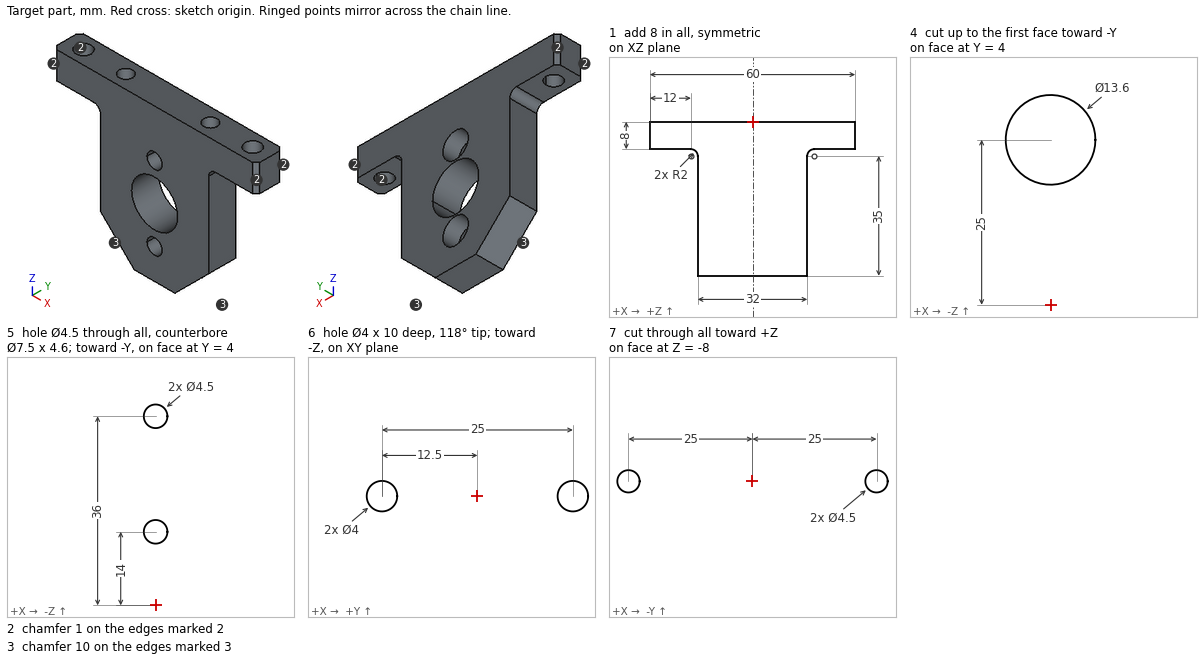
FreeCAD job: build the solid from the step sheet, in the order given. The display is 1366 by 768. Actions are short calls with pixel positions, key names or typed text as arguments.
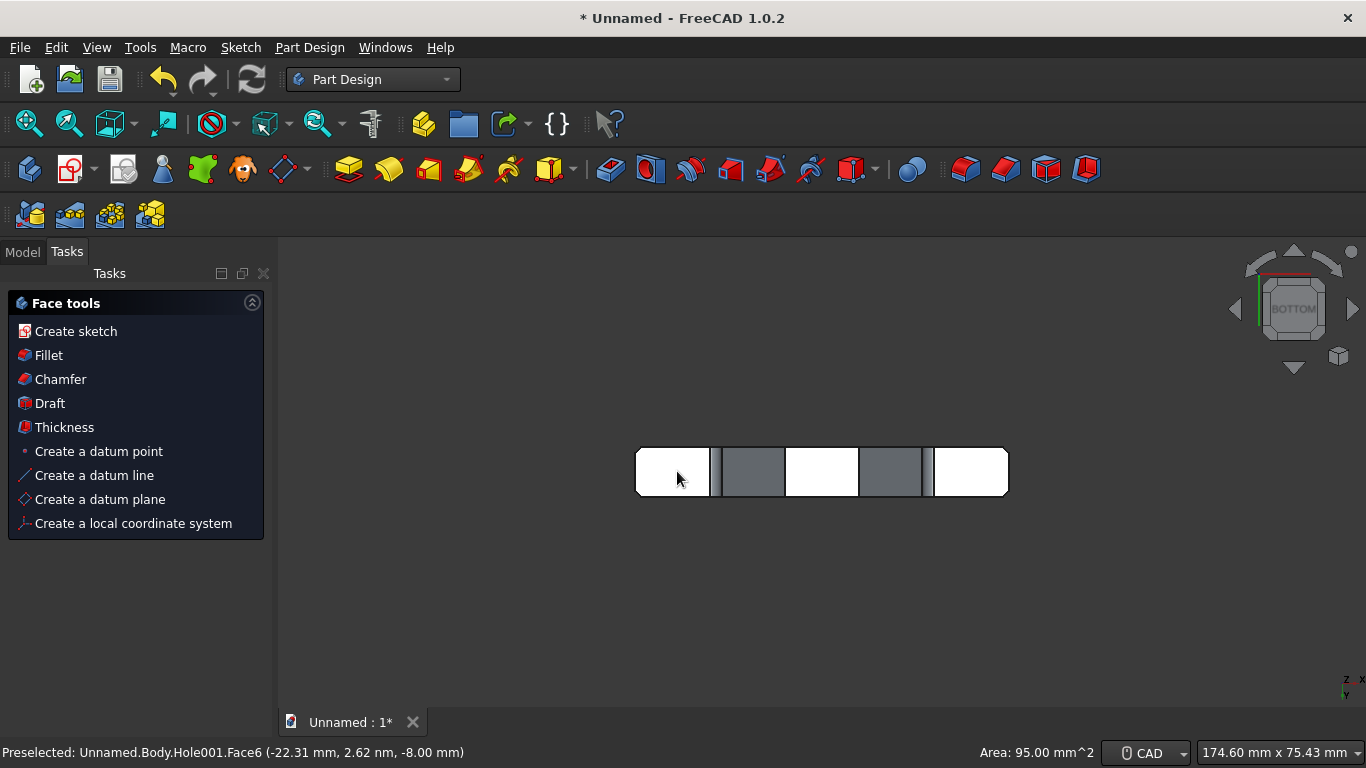
click(70, 170)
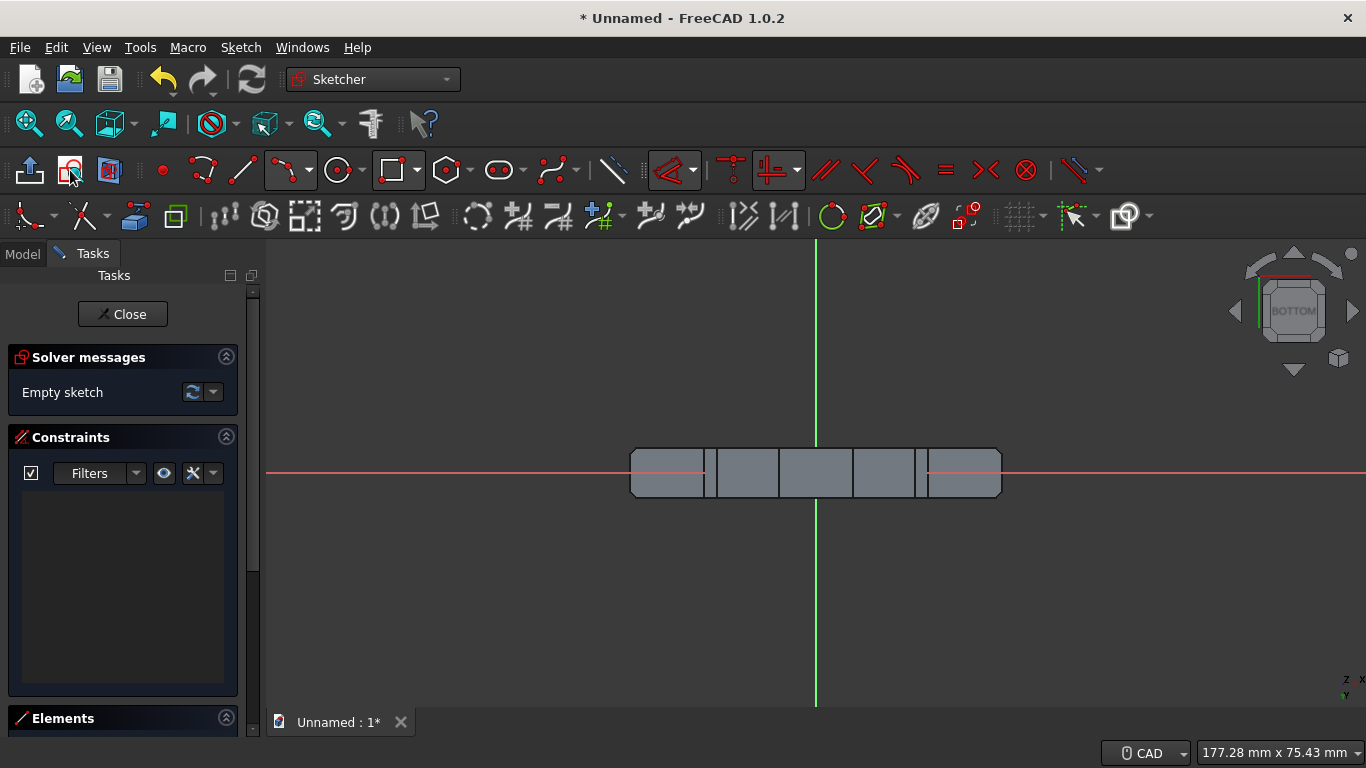
scroll(899, 473, up, 3)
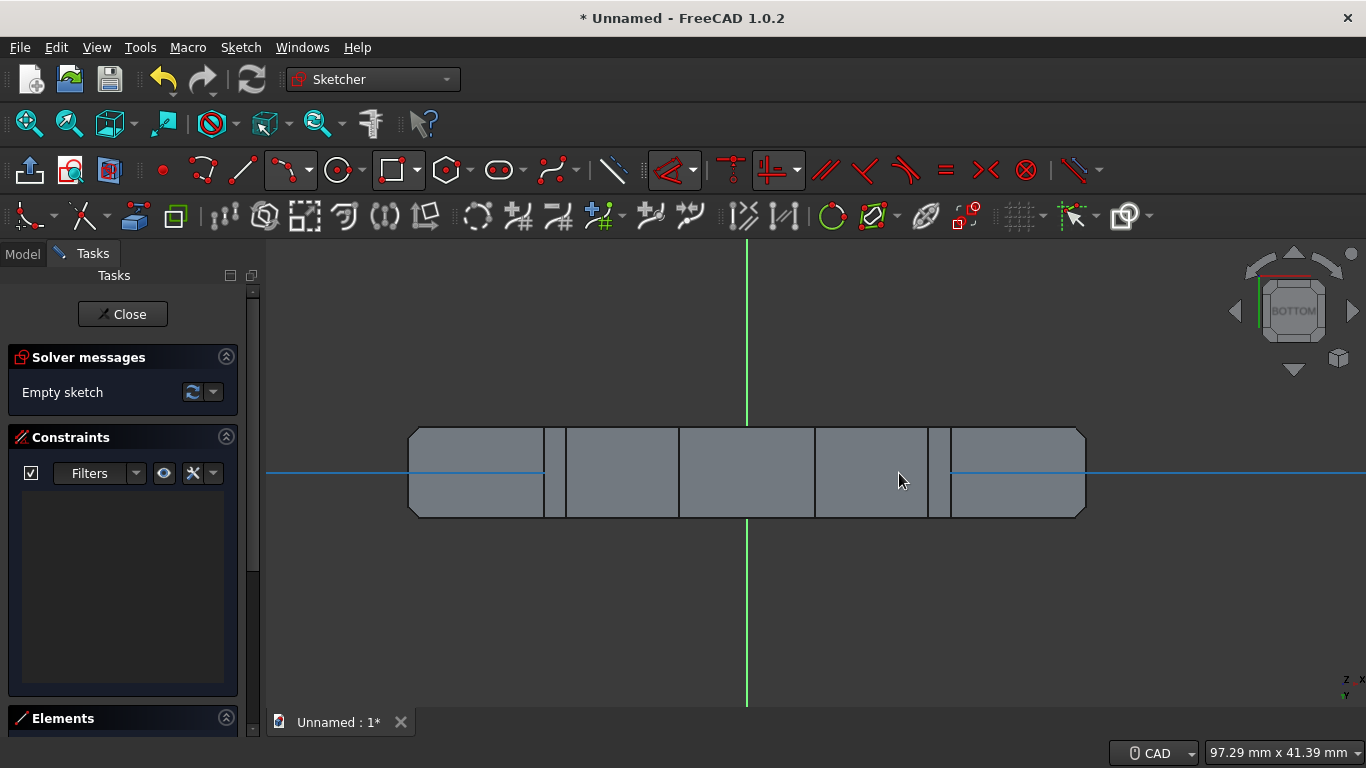
click(338, 170)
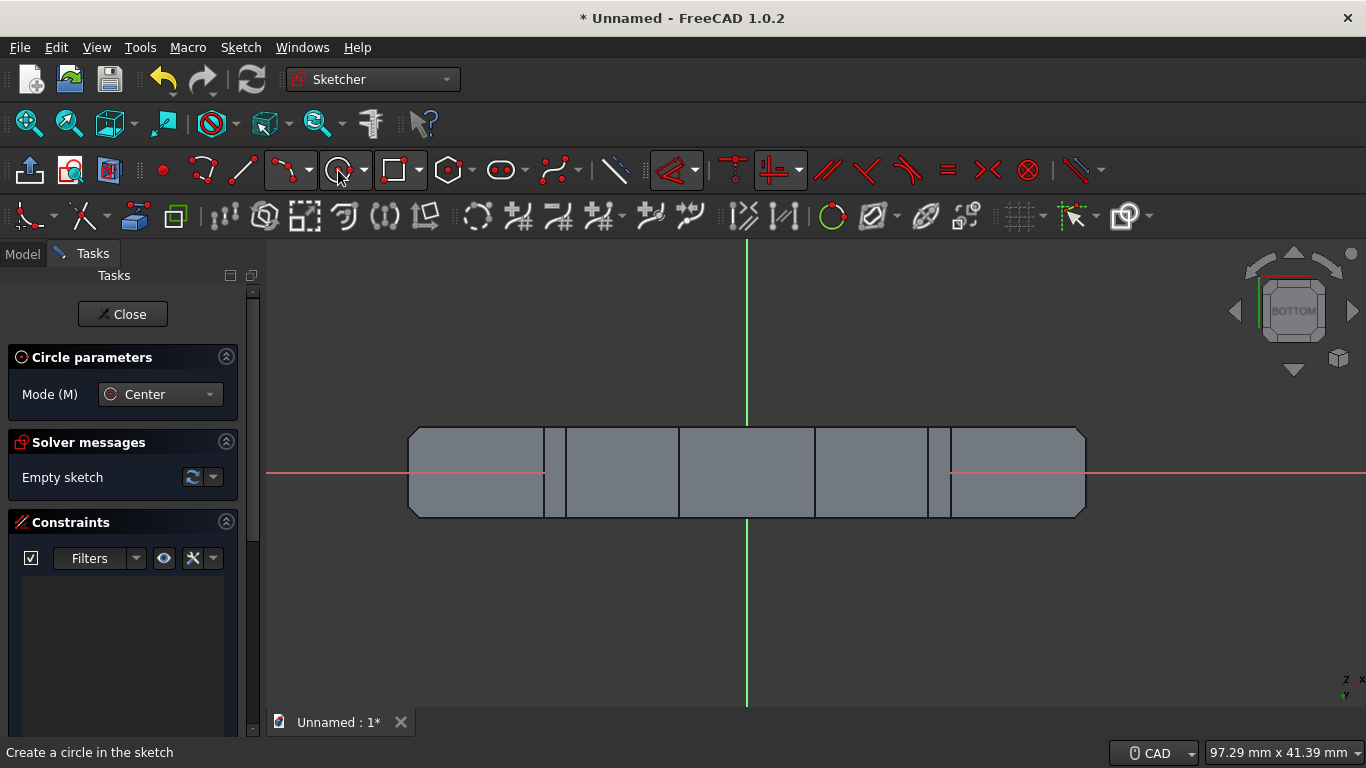
click(1030, 473)
click(1048, 455)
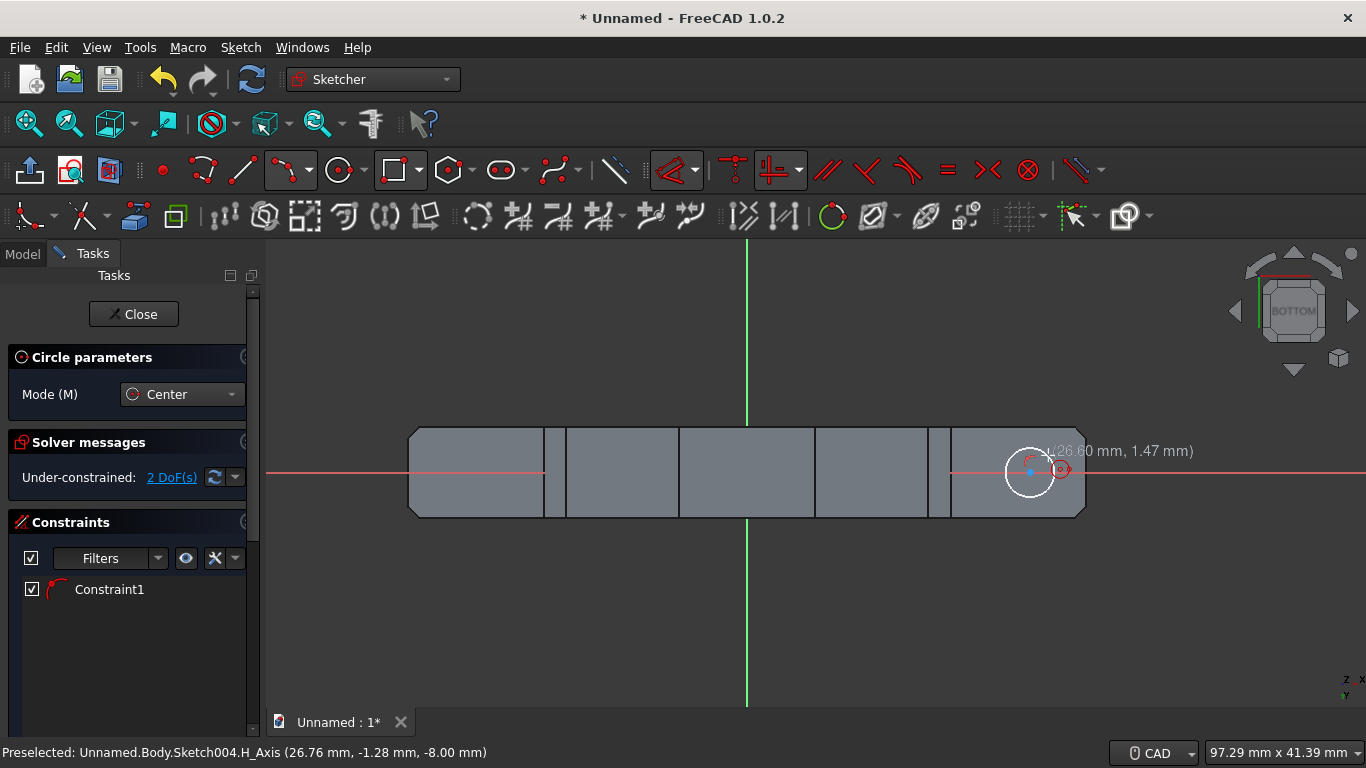
click(465, 473)
click(483, 455)
key(Escape)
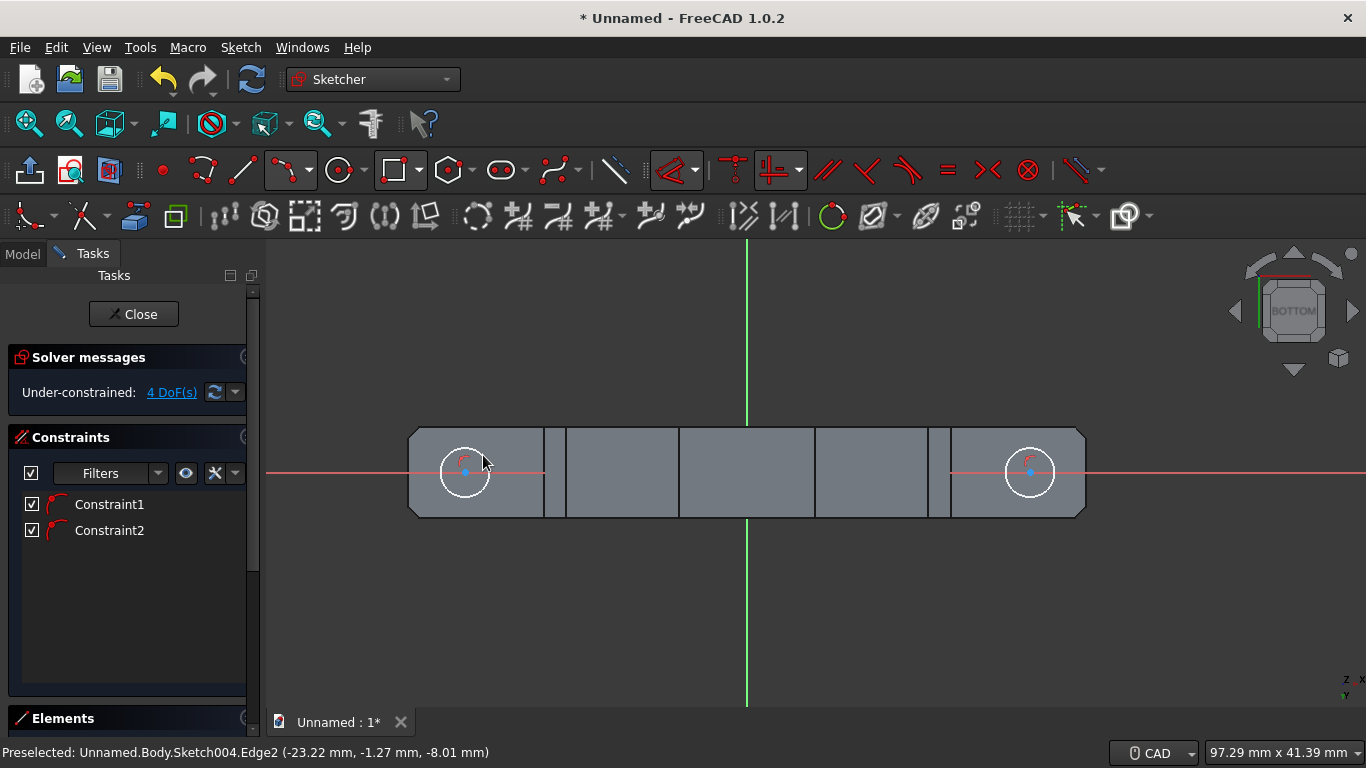
click(1047, 455)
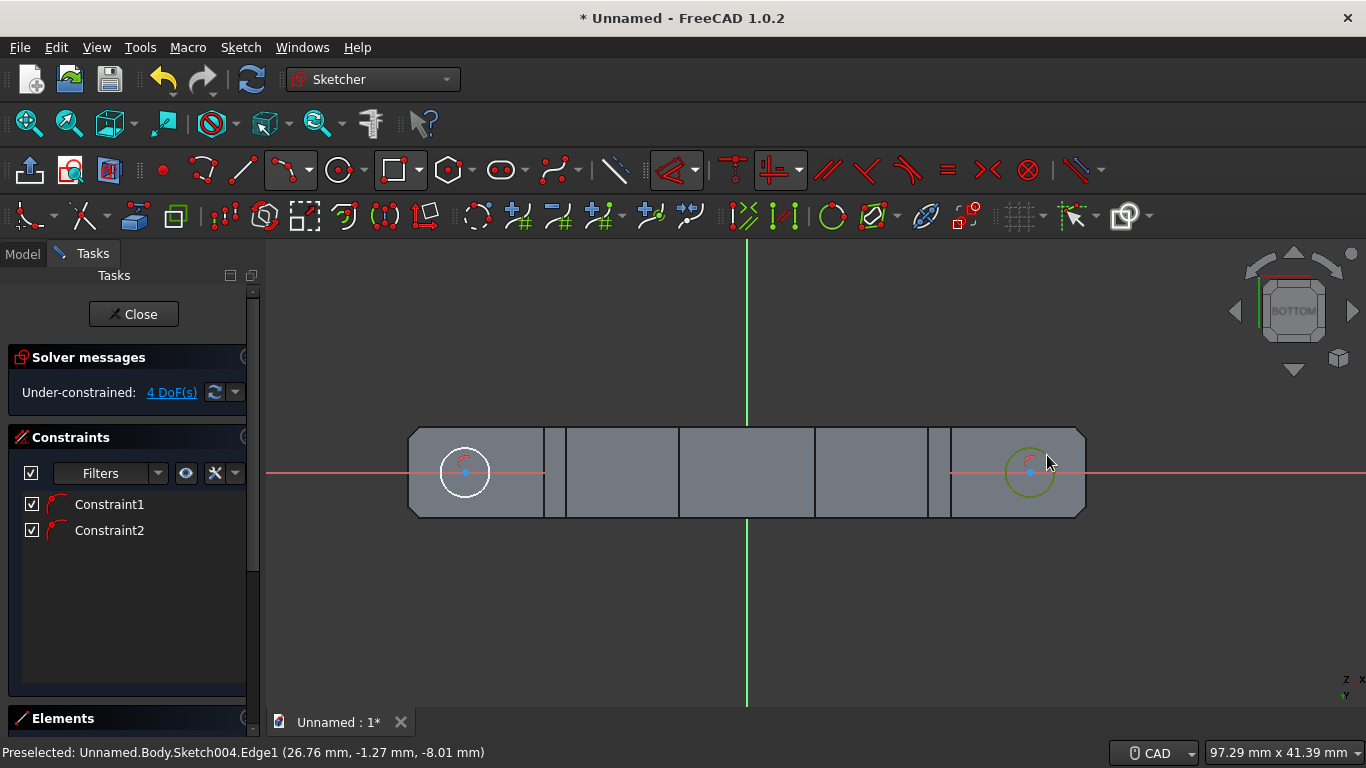
click(482, 455)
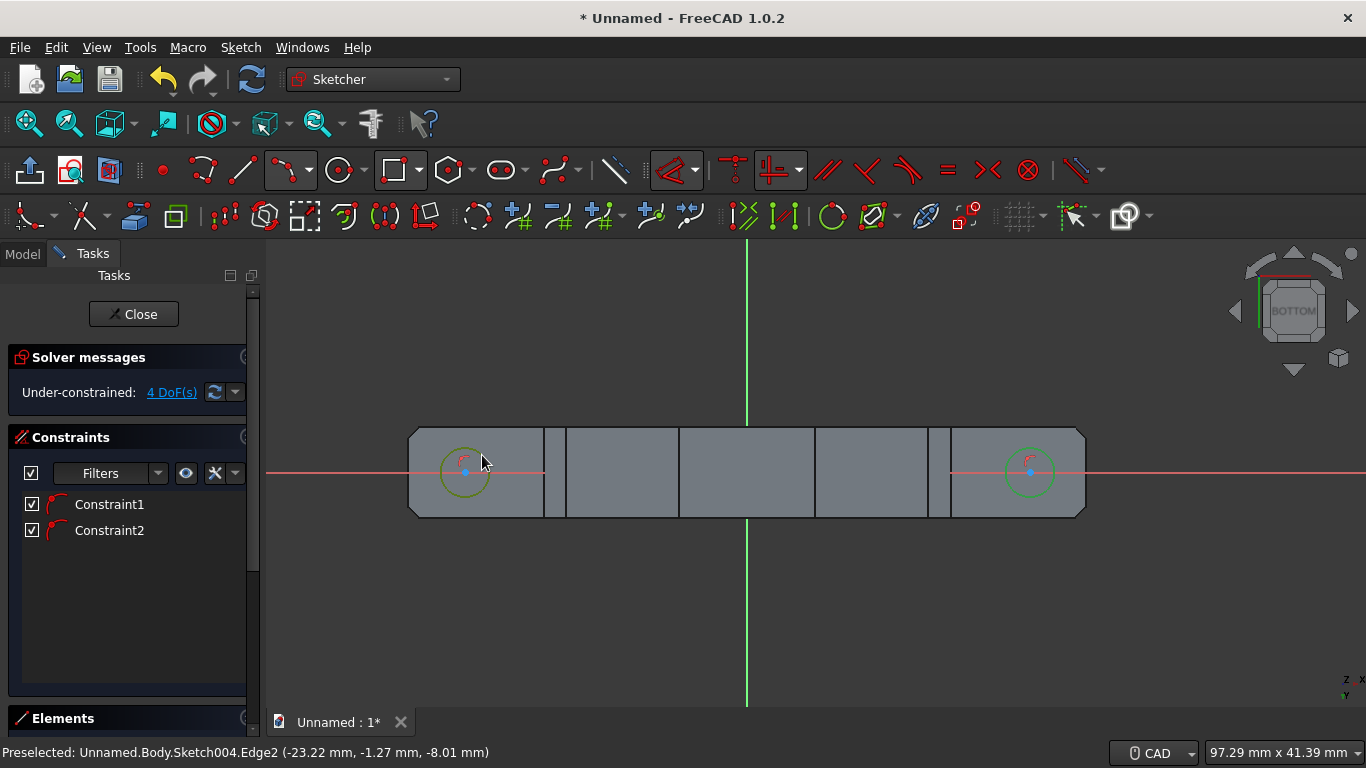
click(948, 170)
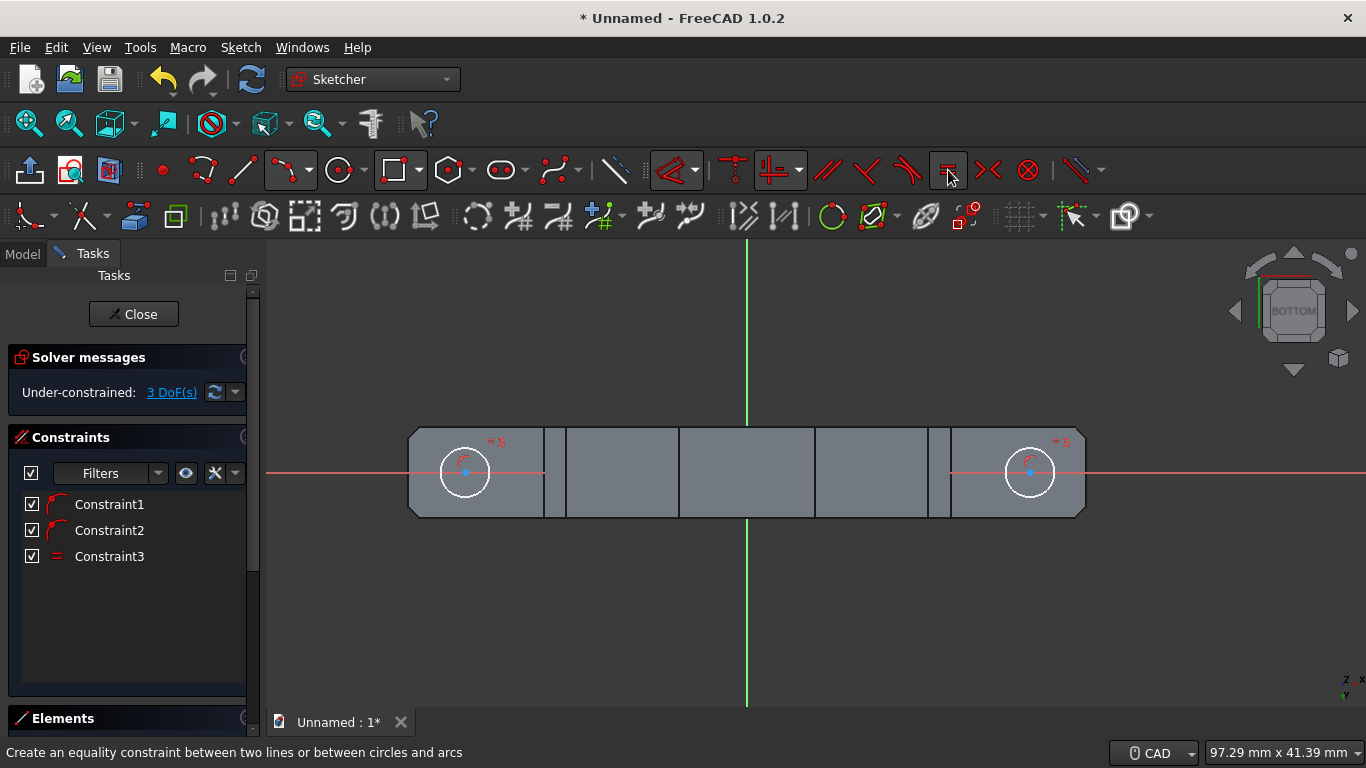
click(1047, 455)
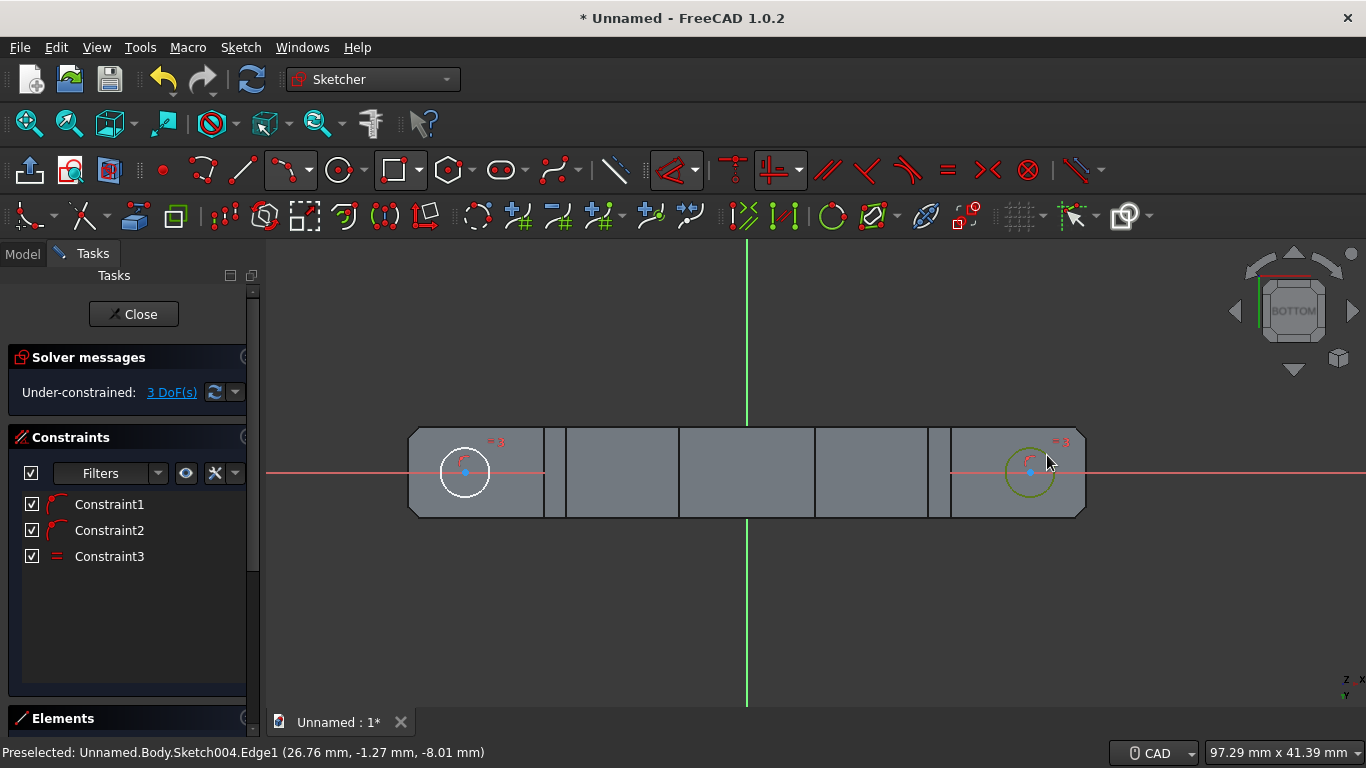
key(k)
key(o)